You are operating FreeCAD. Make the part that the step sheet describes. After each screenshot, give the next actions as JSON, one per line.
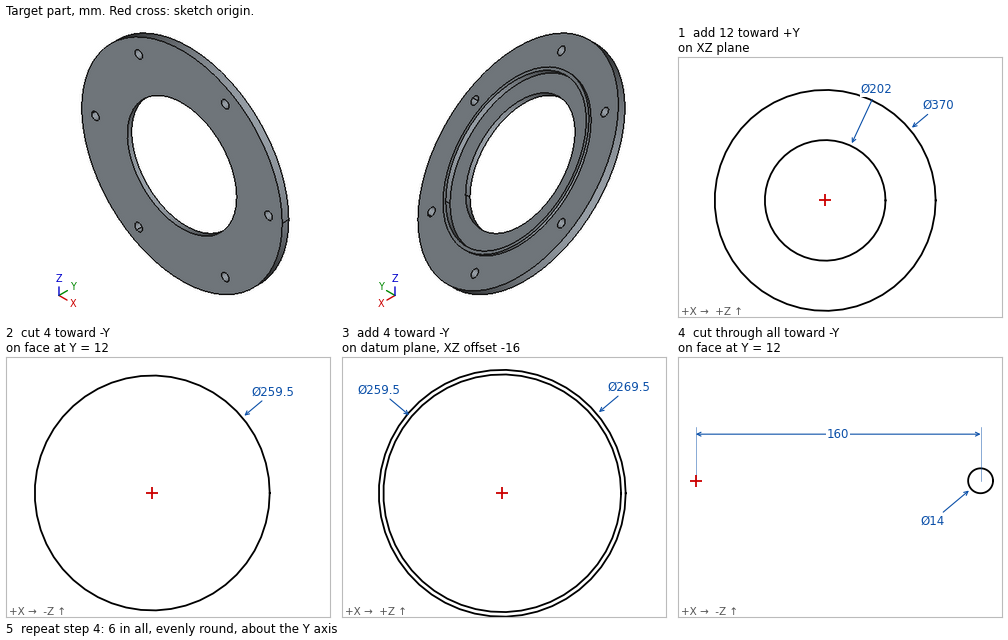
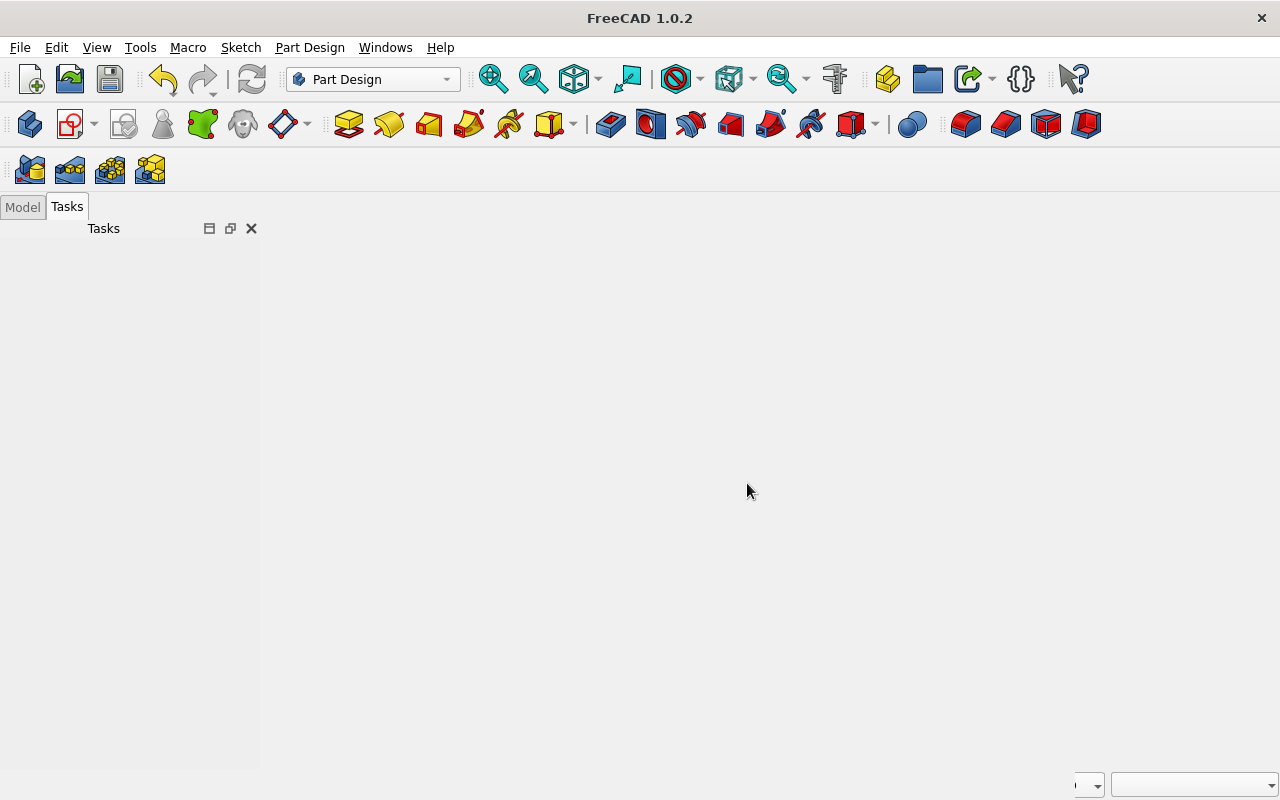
{"action": "left_click", "coordinate": [30, 80]}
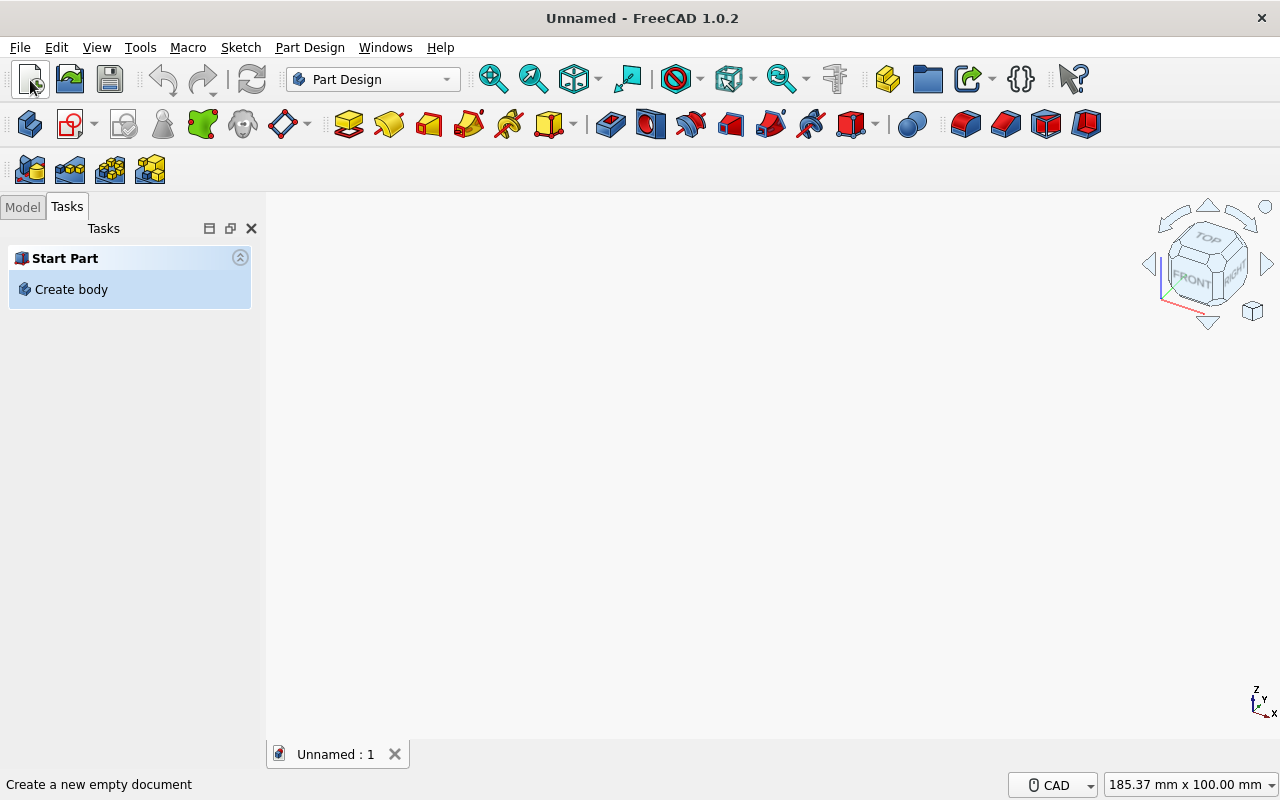
{"action": "left_click", "coordinate": [70, 124]}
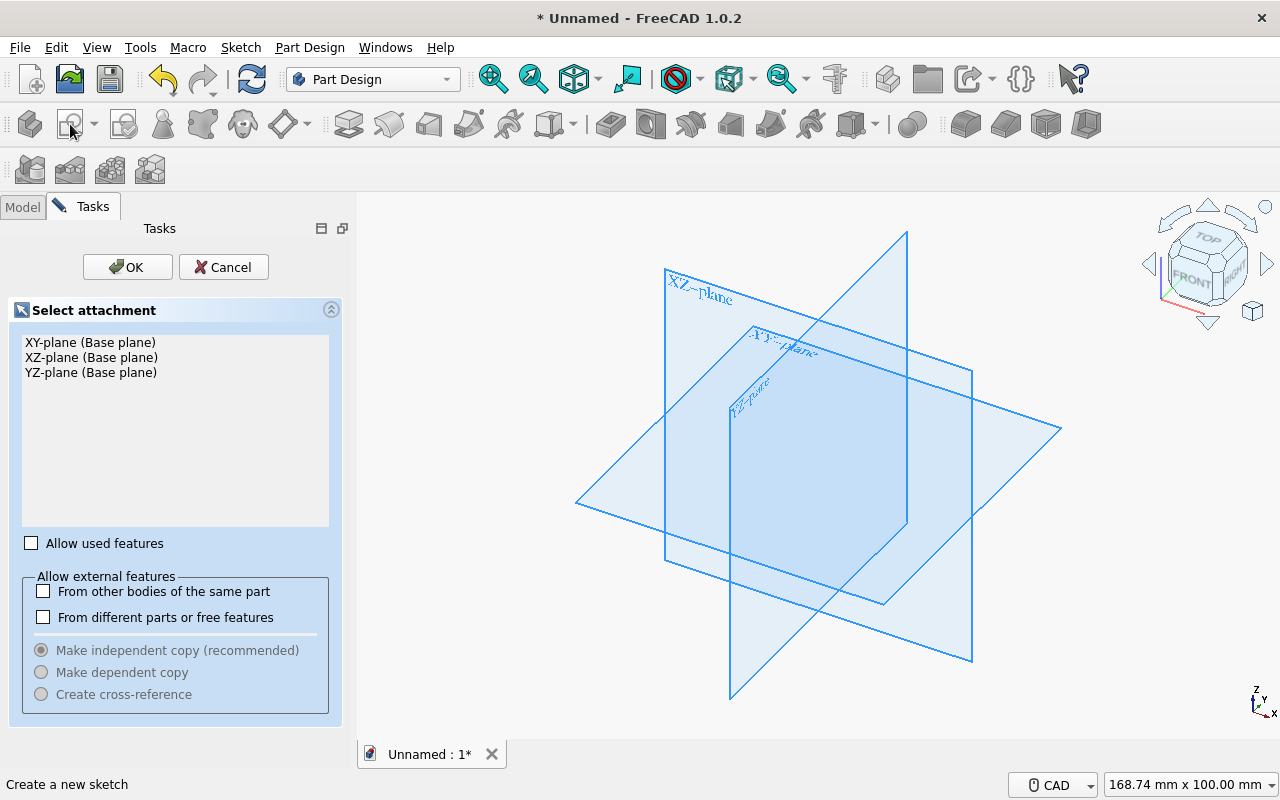
{"action": "left_click", "coordinate": [82, 358]}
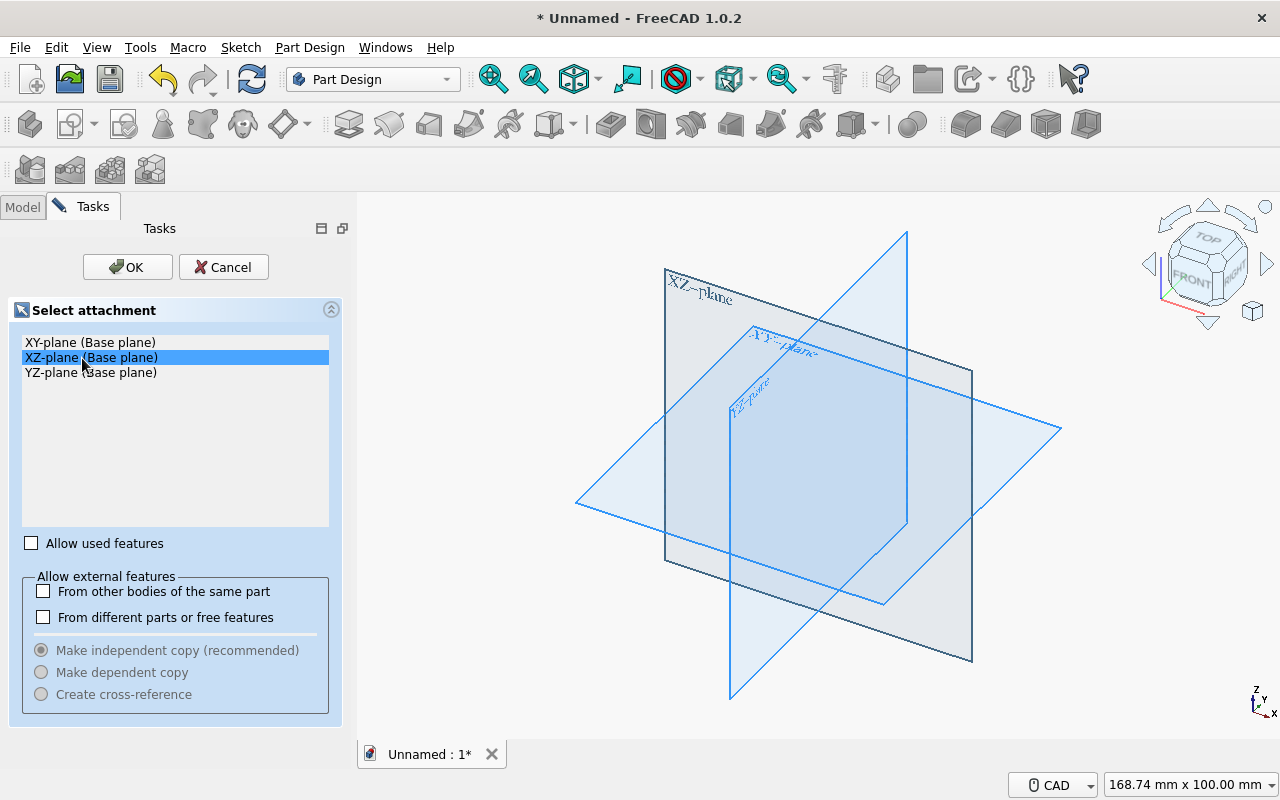
{"action": "left_click", "coordinate": [128, 267]}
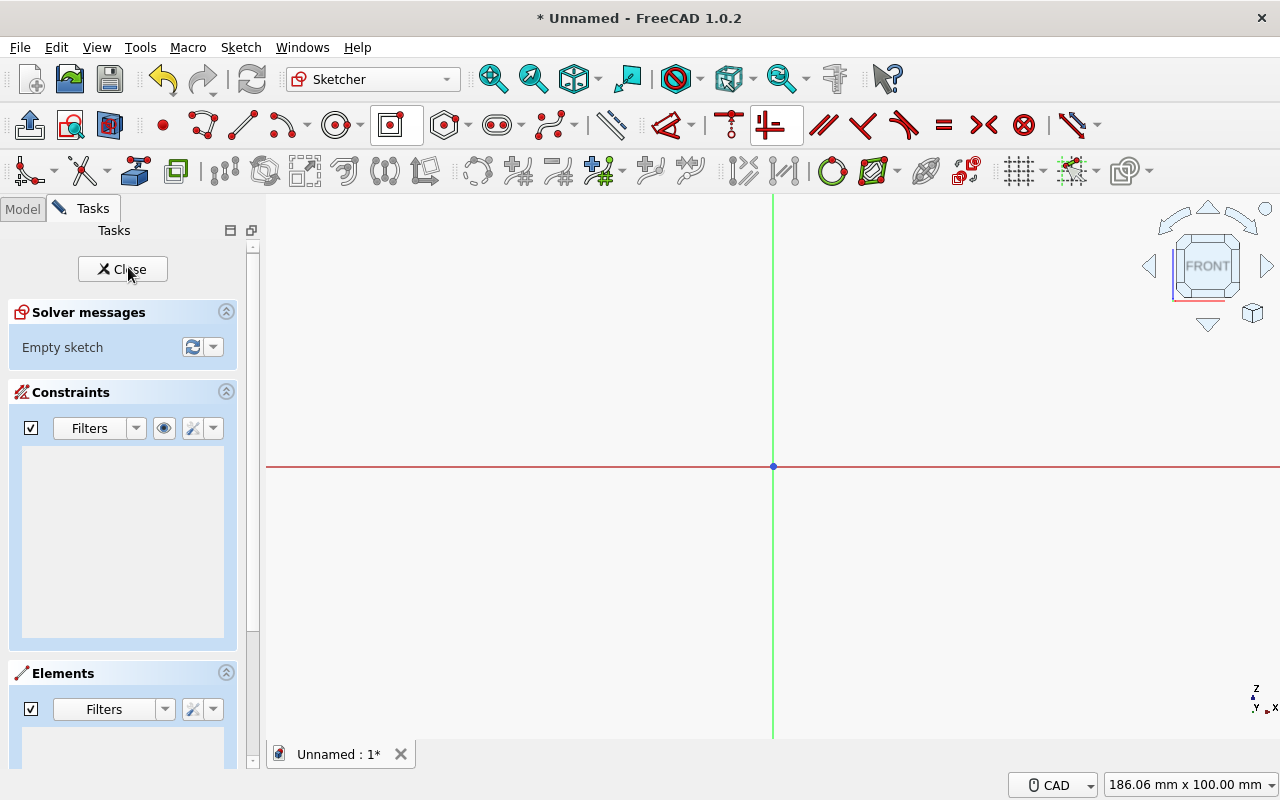
{"action": "scroll", "coordinate": [691, 466], "scroll_direction": "down", "scroll_amount": 9}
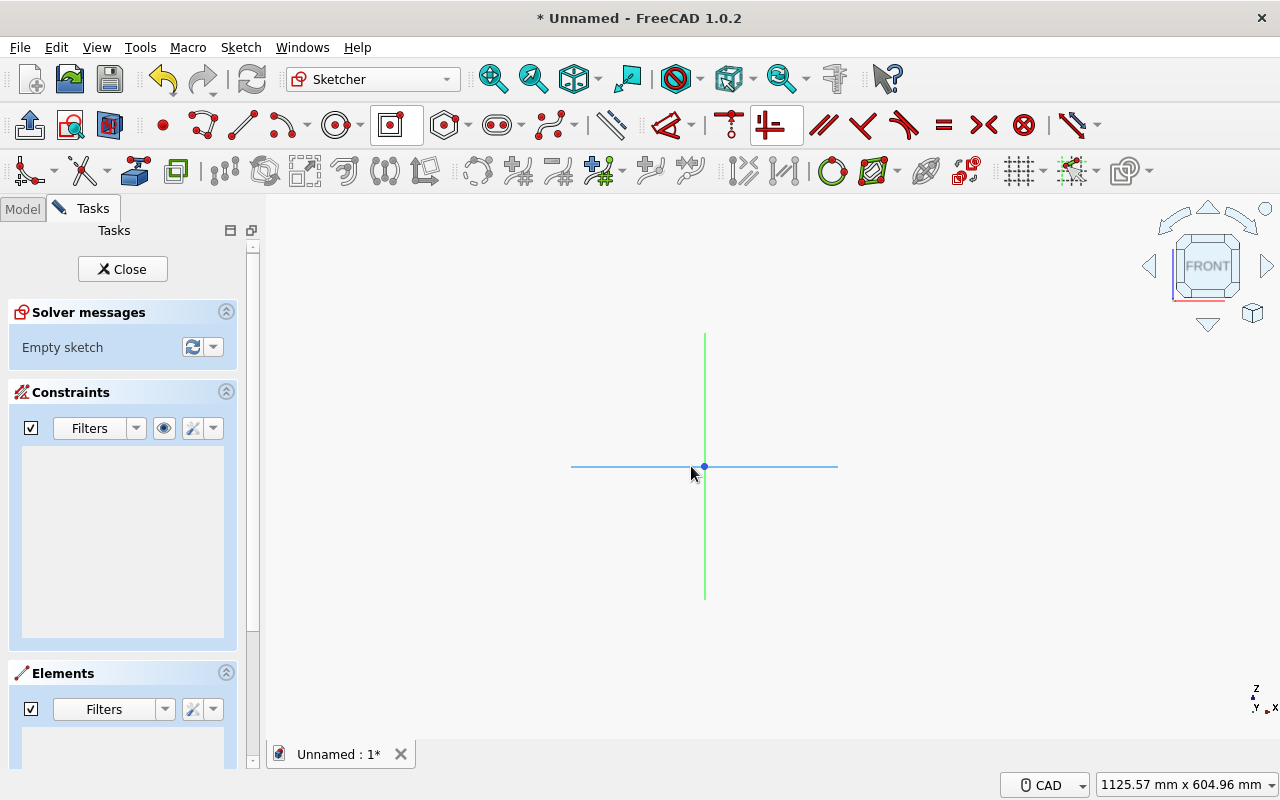
{"action": "left_click", "coordinate": [336, 126]}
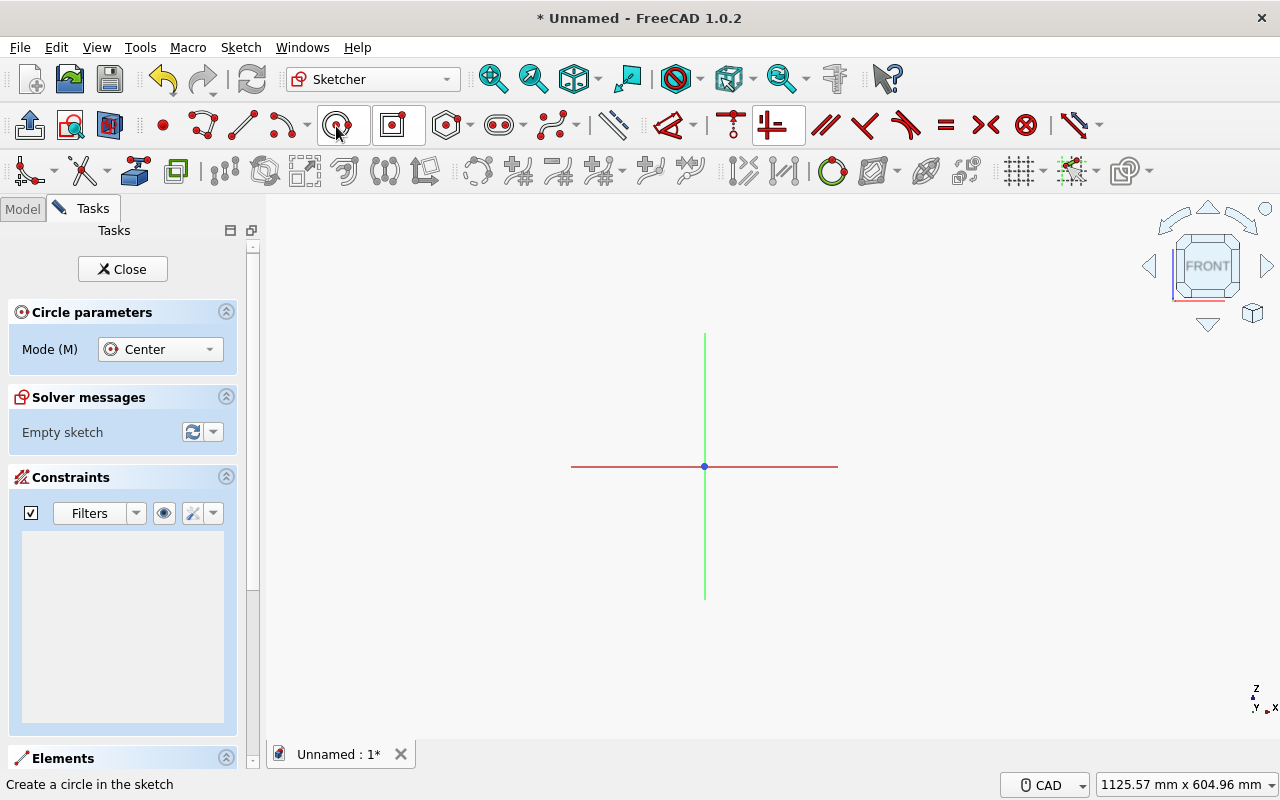
{"action": "left_click", "coordinate": [705, 466]}
{"action": "mouse_move", "coordinate": [823, 349]}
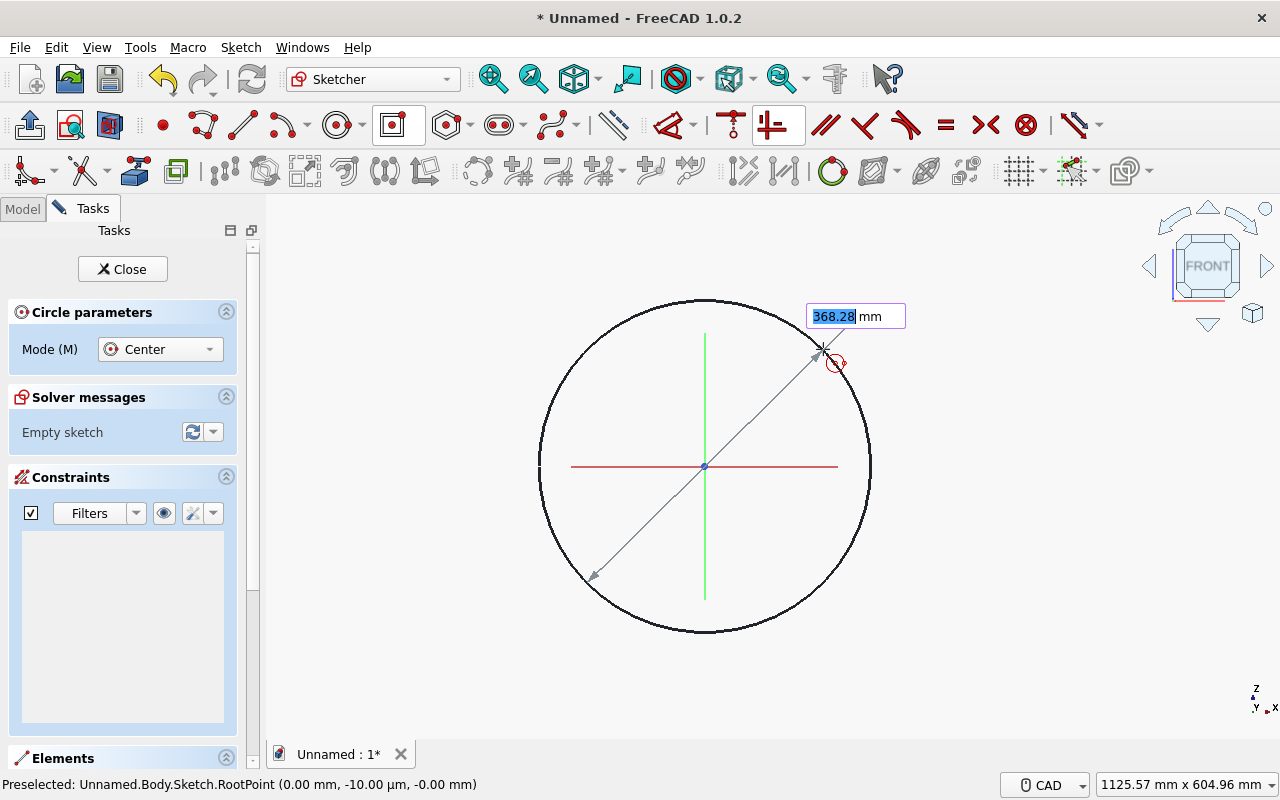
{"action": "type", "text": "370"}
{"action": "key", "text": "Return"}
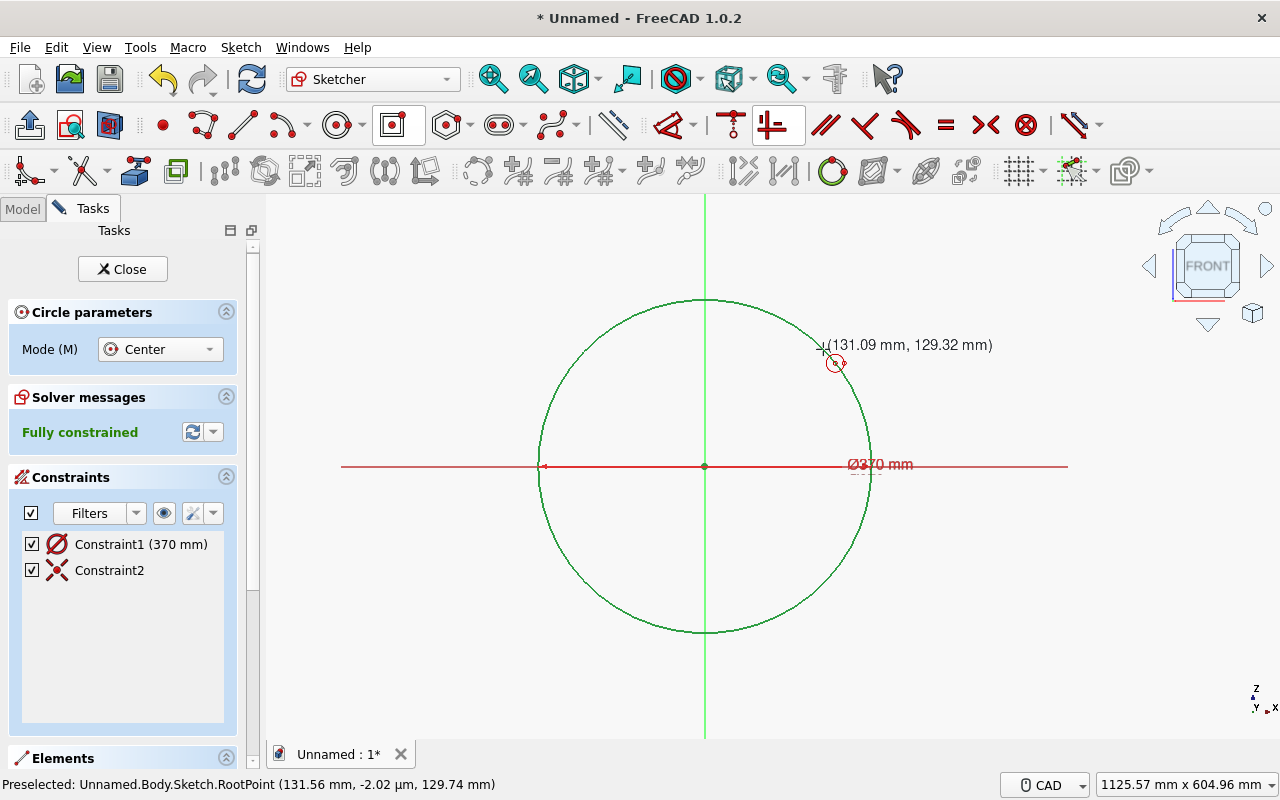
{"action": "left_click", "coordinate": [705, 466]}
{"action": "mouse_move", "coordinate": [769, 402]}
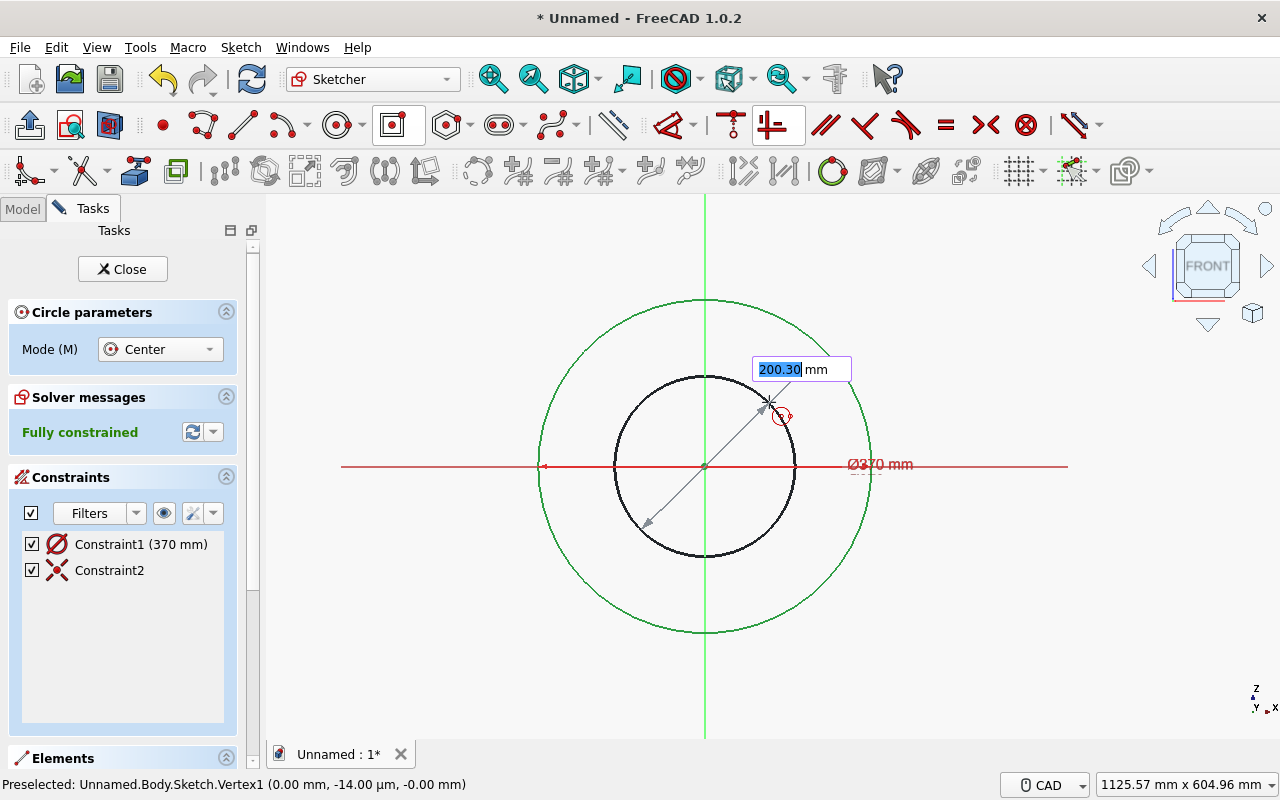
{"action": "type", "text": "202"}
{"action": "key", "text": "Return"}
{"action": "key", "text": "Escape"}